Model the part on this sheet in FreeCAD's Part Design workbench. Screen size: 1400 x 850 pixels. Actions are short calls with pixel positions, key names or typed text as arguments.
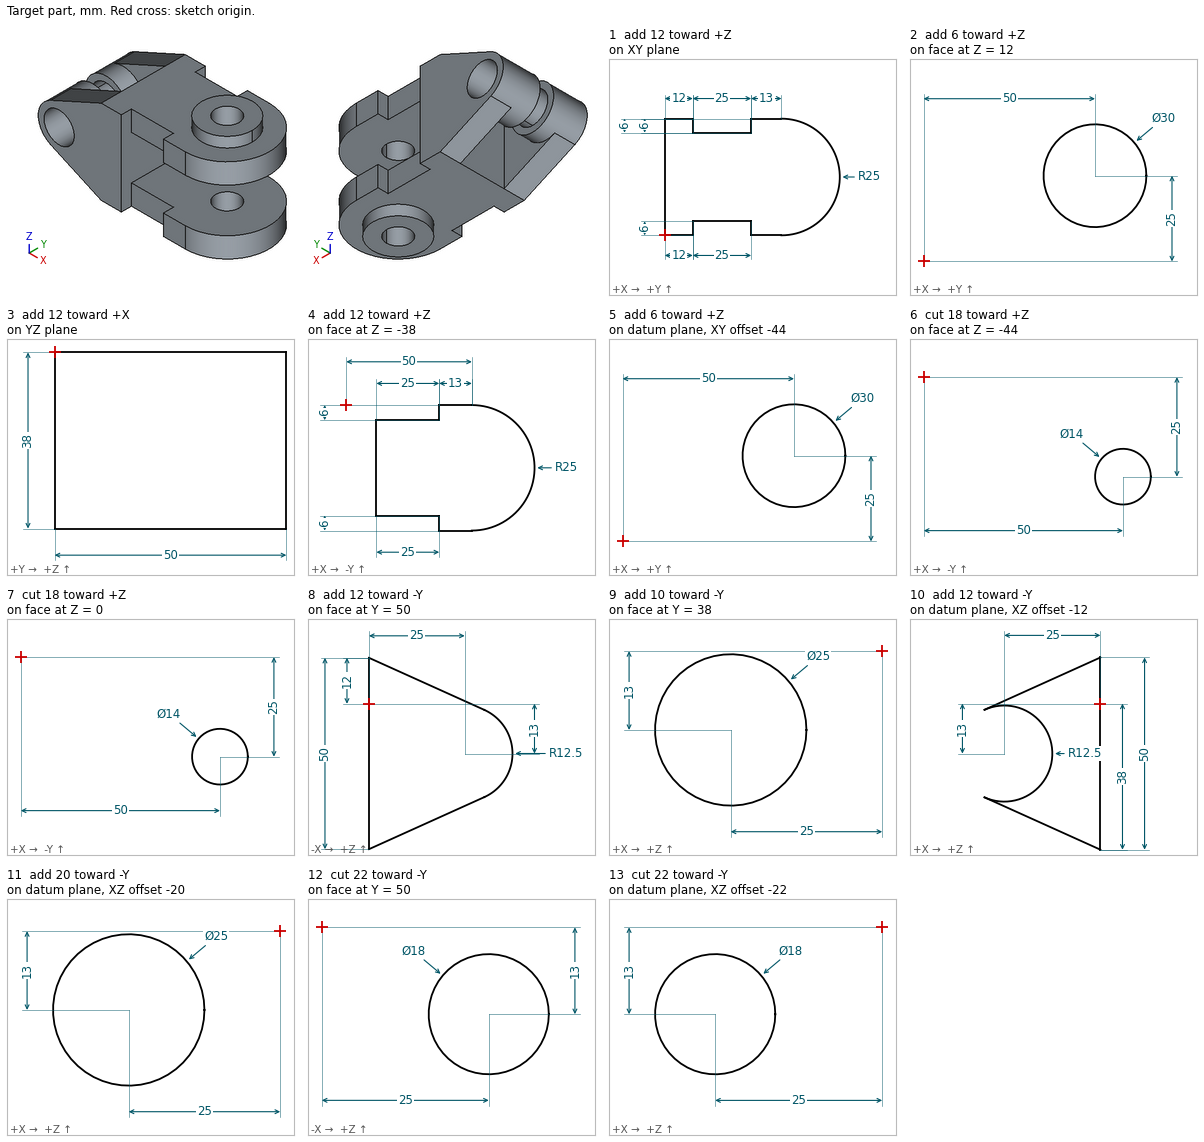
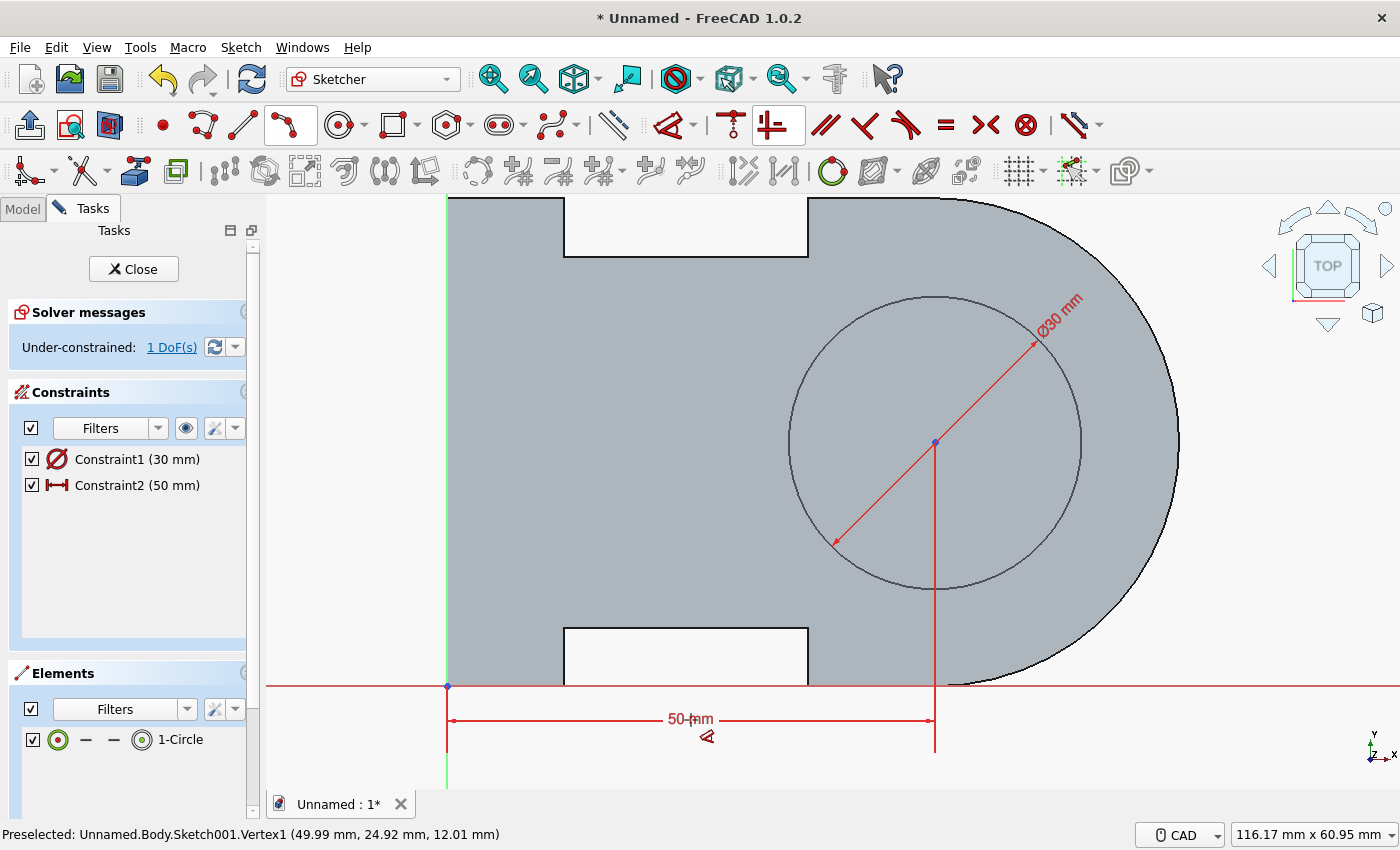
click(935, 443)
click(413, 565)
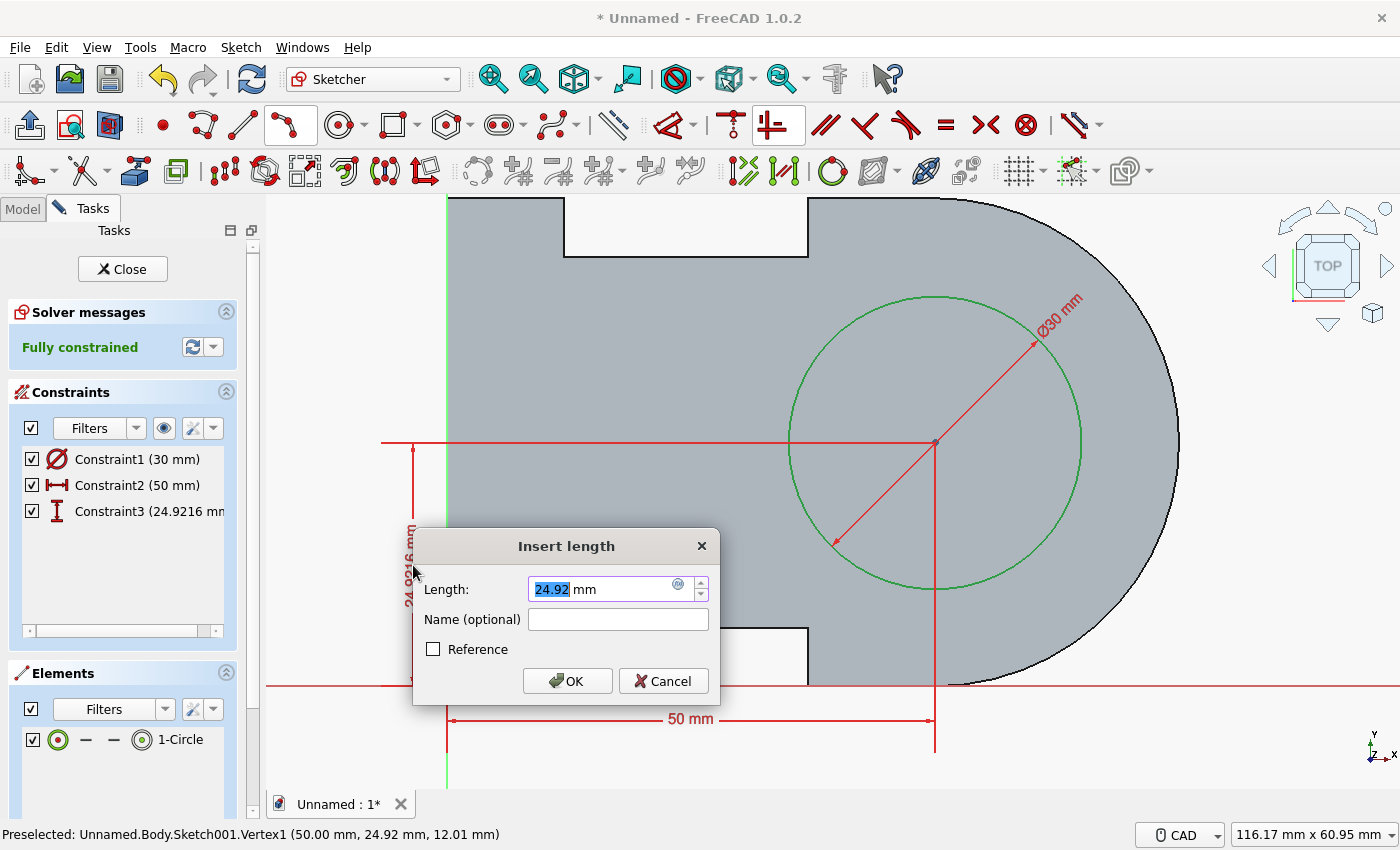
text(25)
key(Return)
key(Escape)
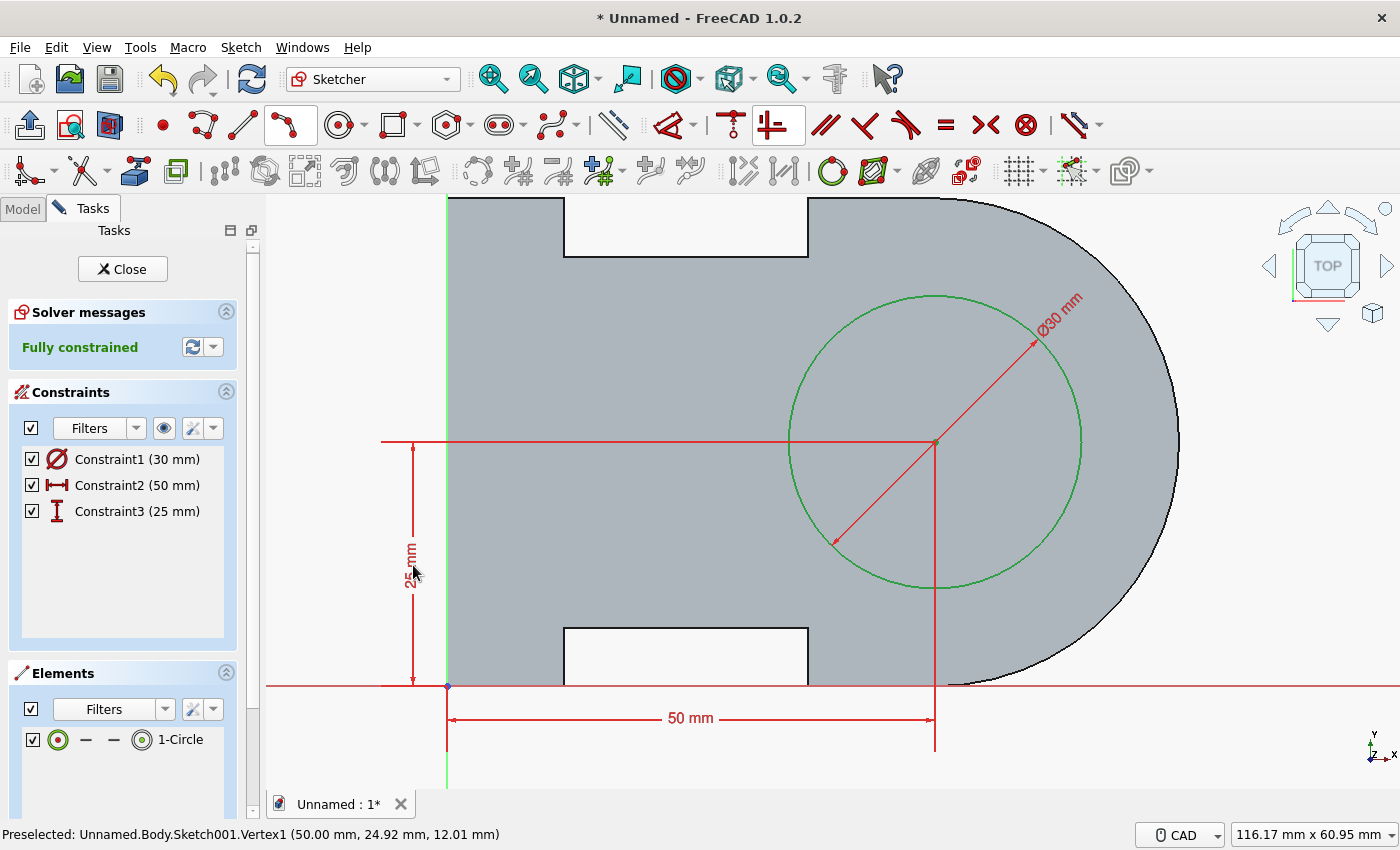
click(123, 269)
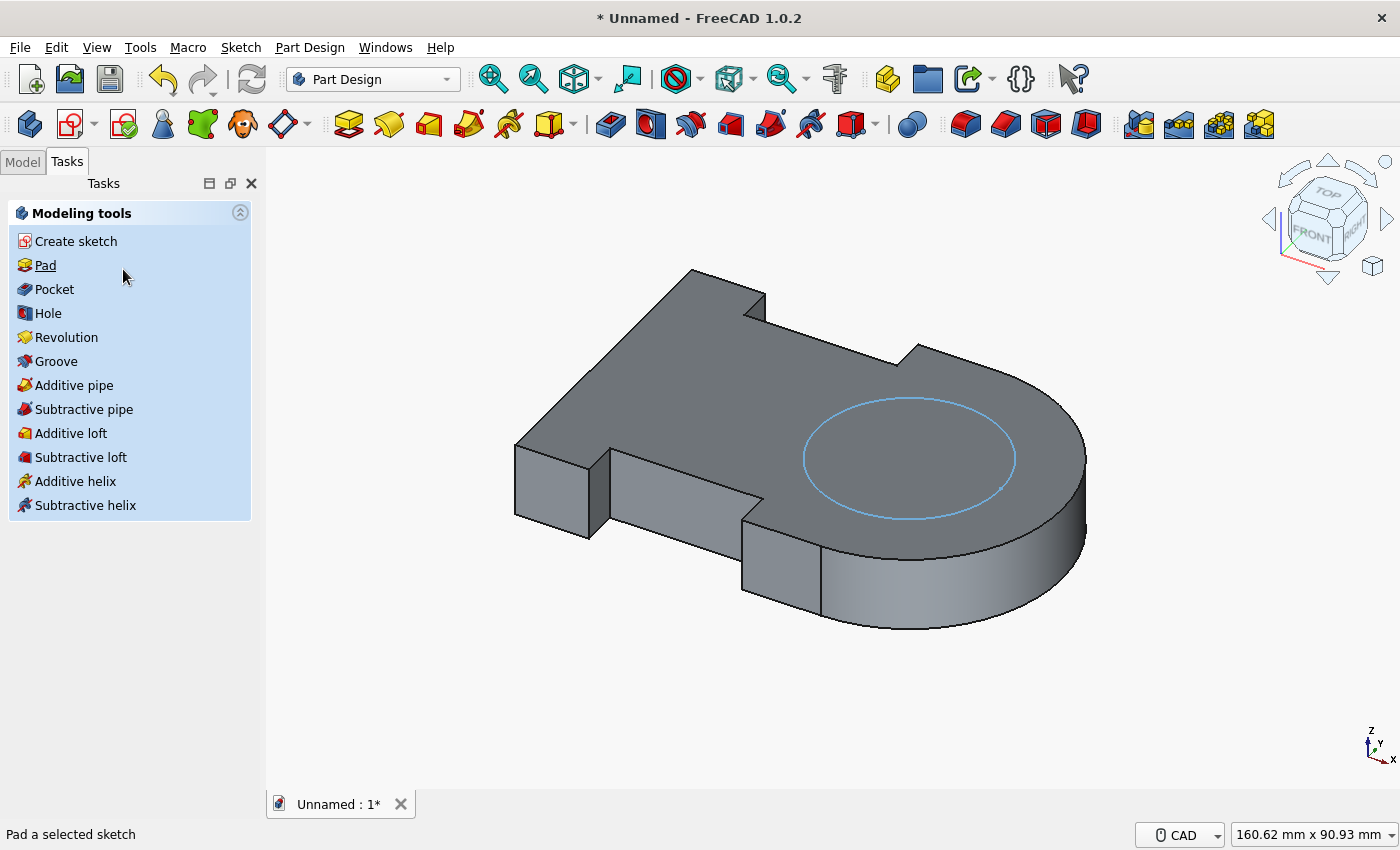
click(350, 124)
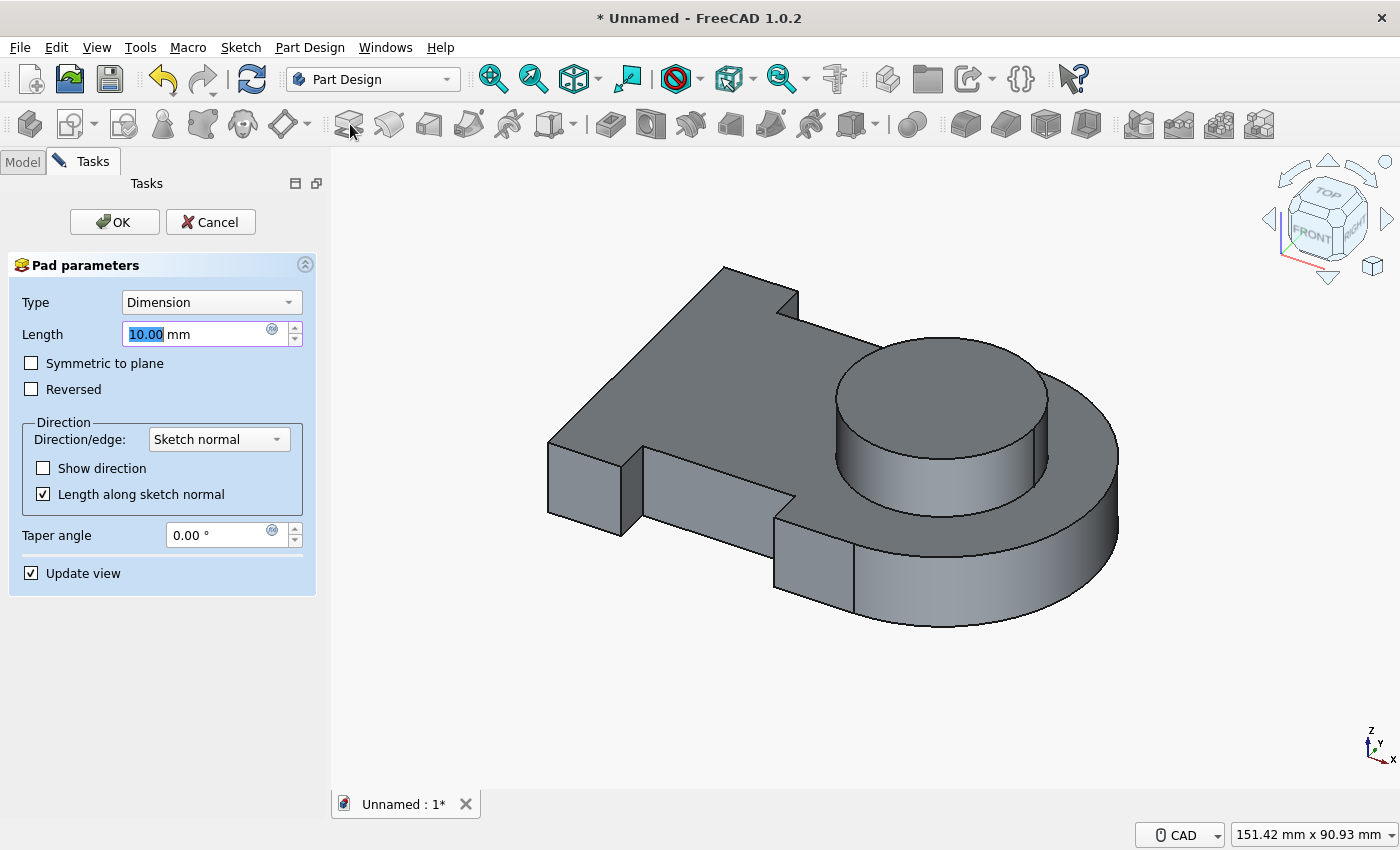
text(6)
key(Tab)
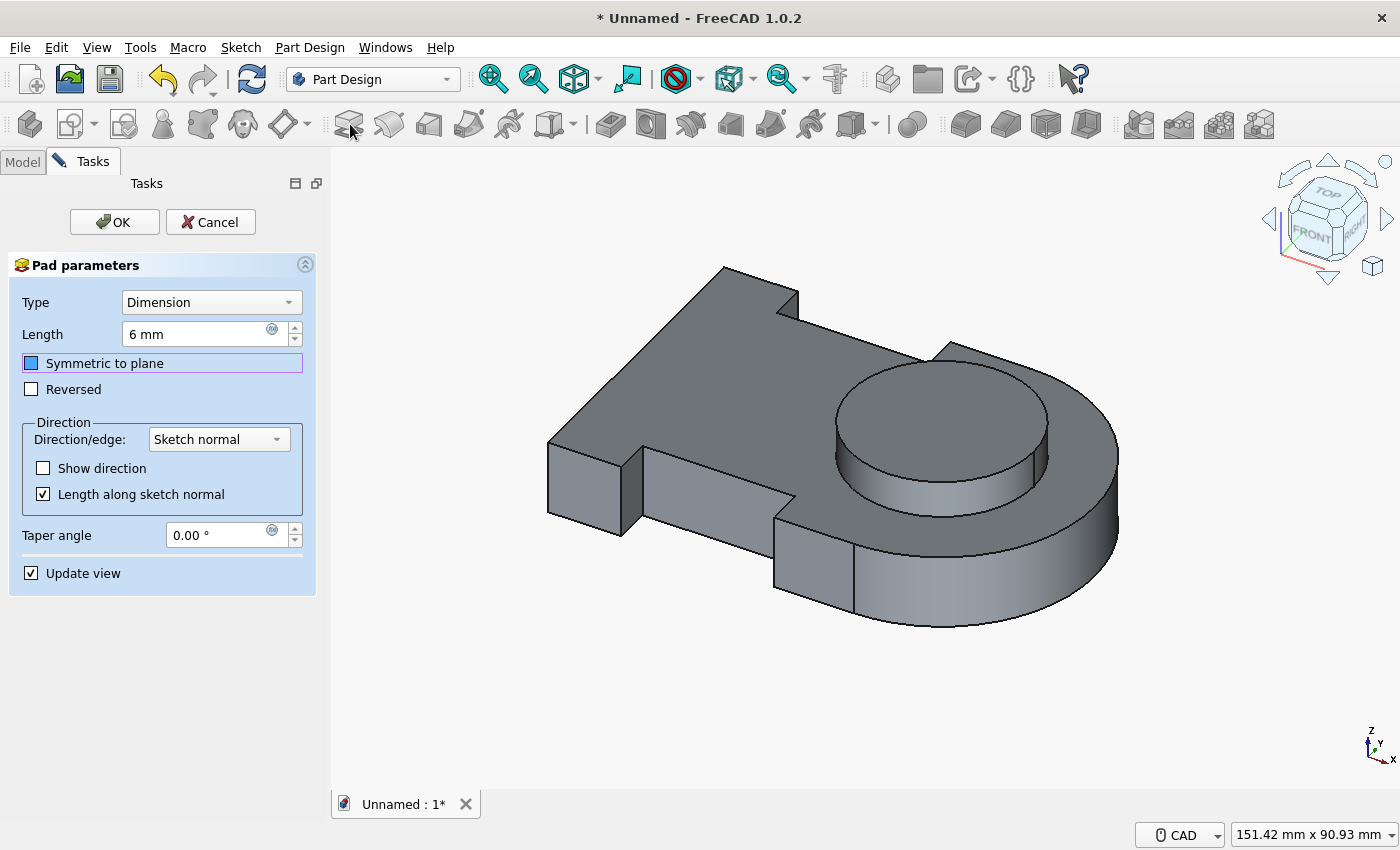
click(115, 222)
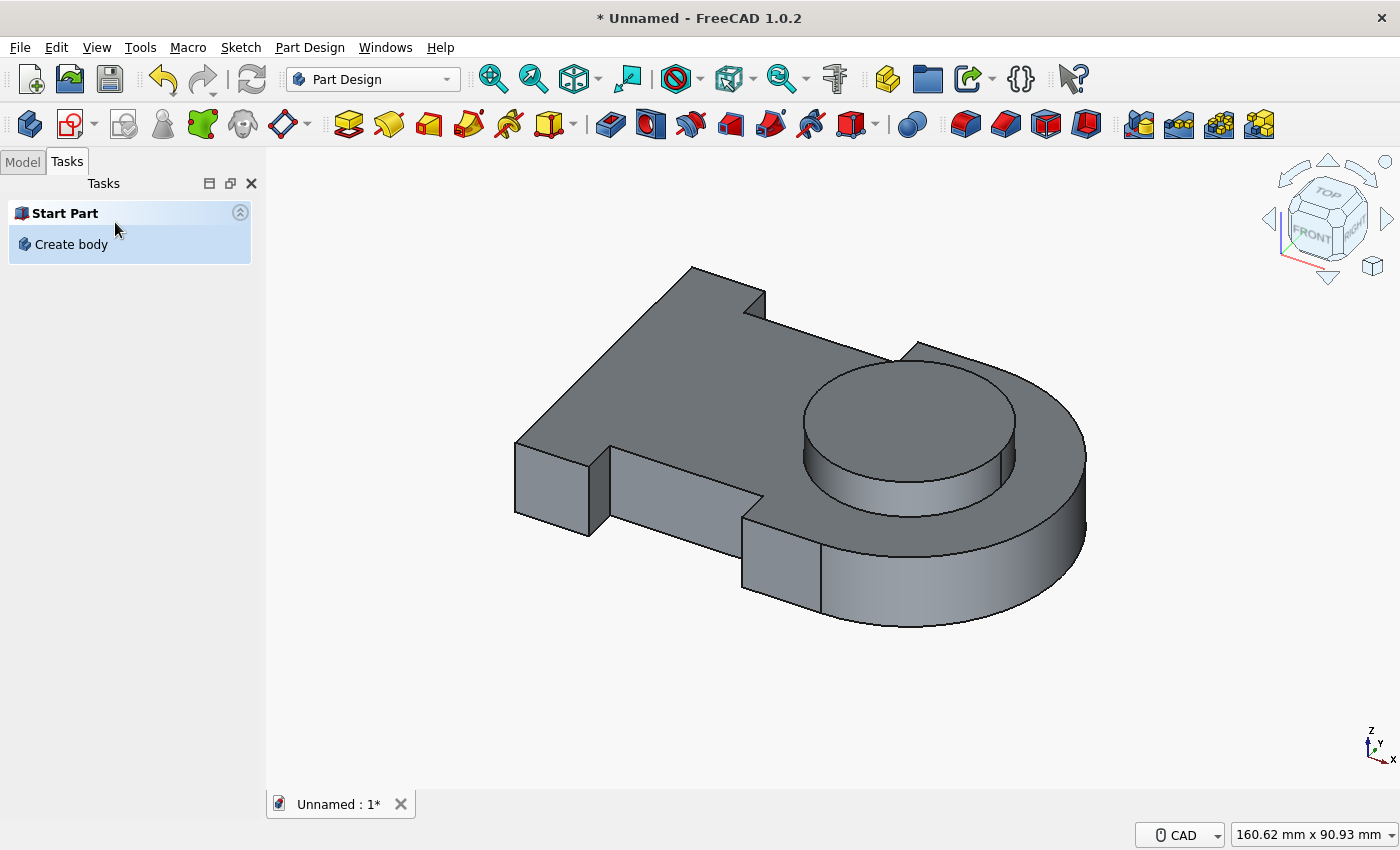
click(70, 124)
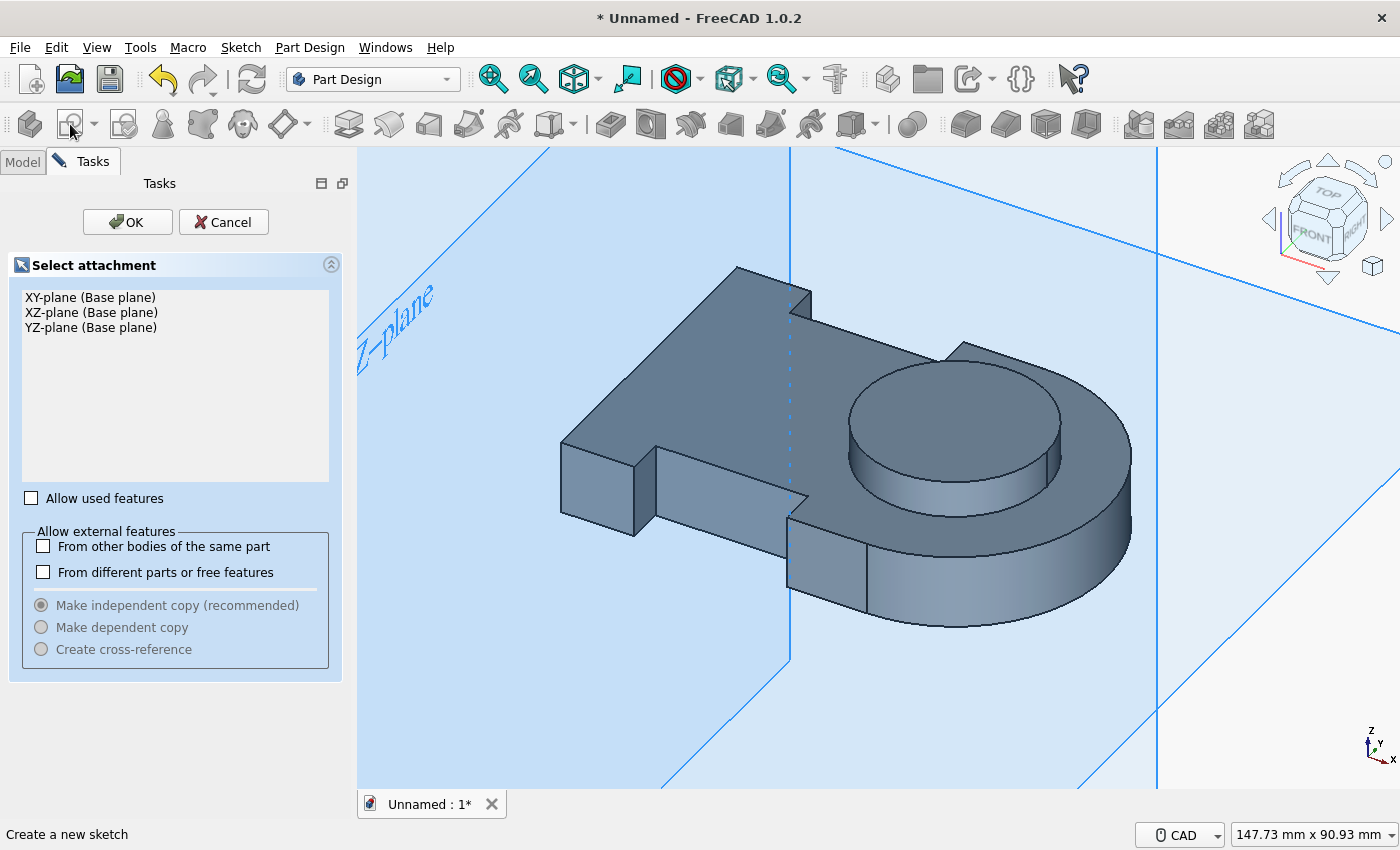
click(82, 328)